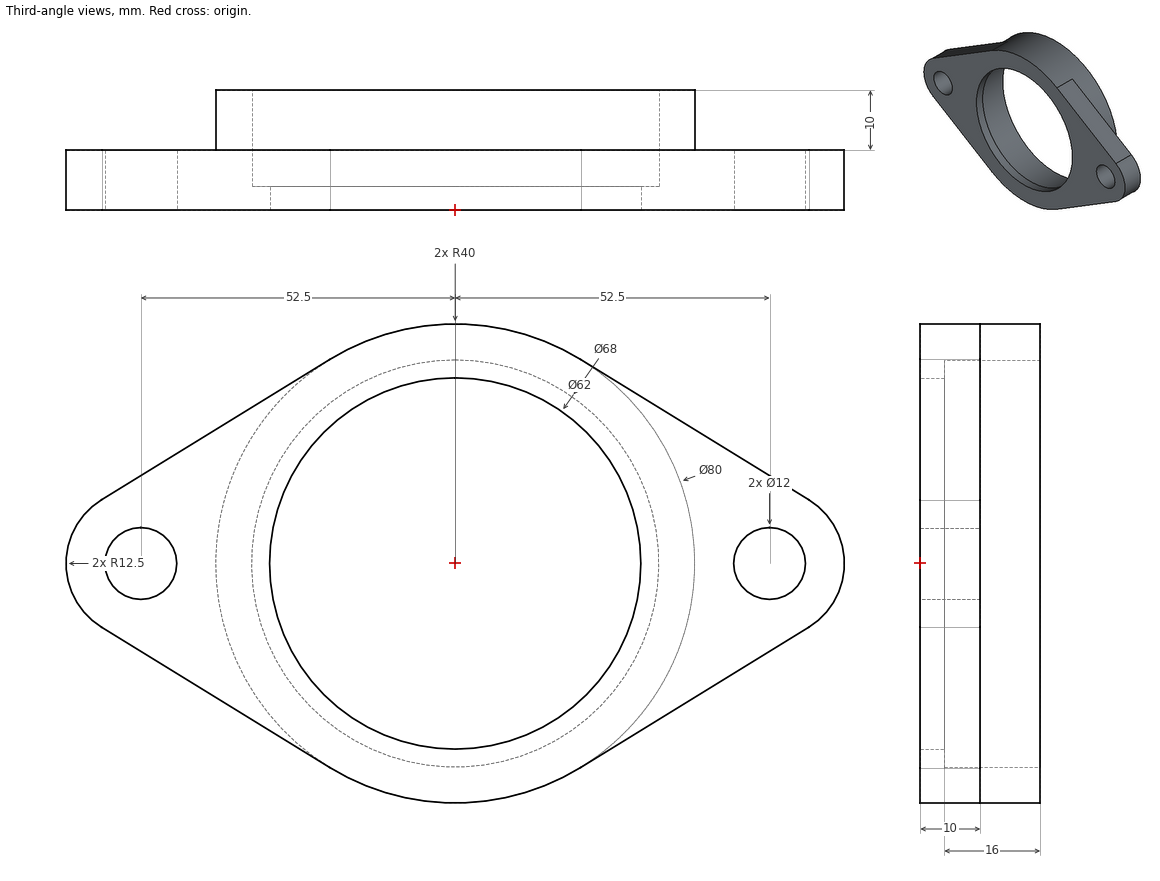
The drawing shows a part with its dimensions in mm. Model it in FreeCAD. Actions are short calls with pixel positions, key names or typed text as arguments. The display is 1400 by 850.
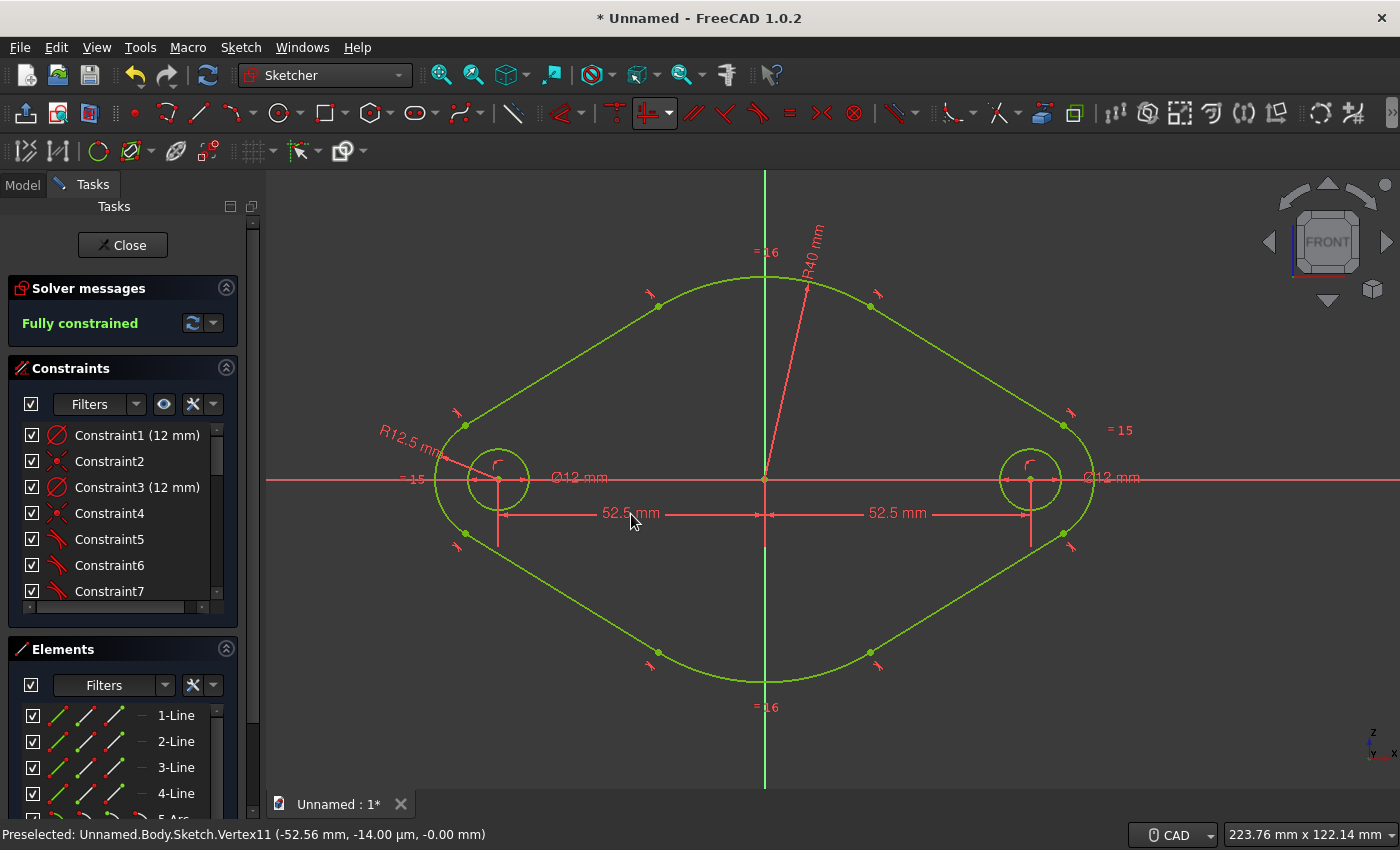
click(123, 245)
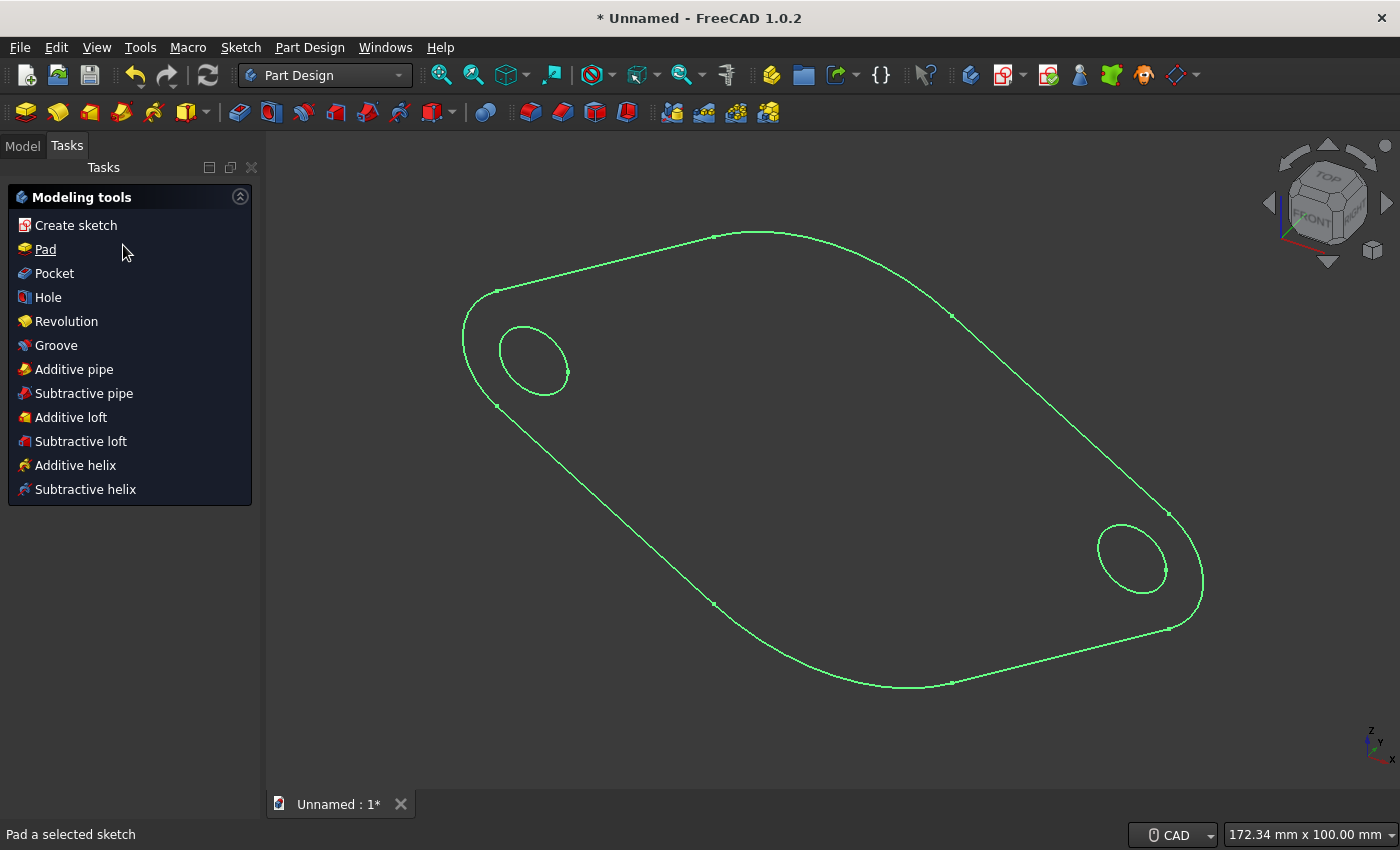
click(26, 112)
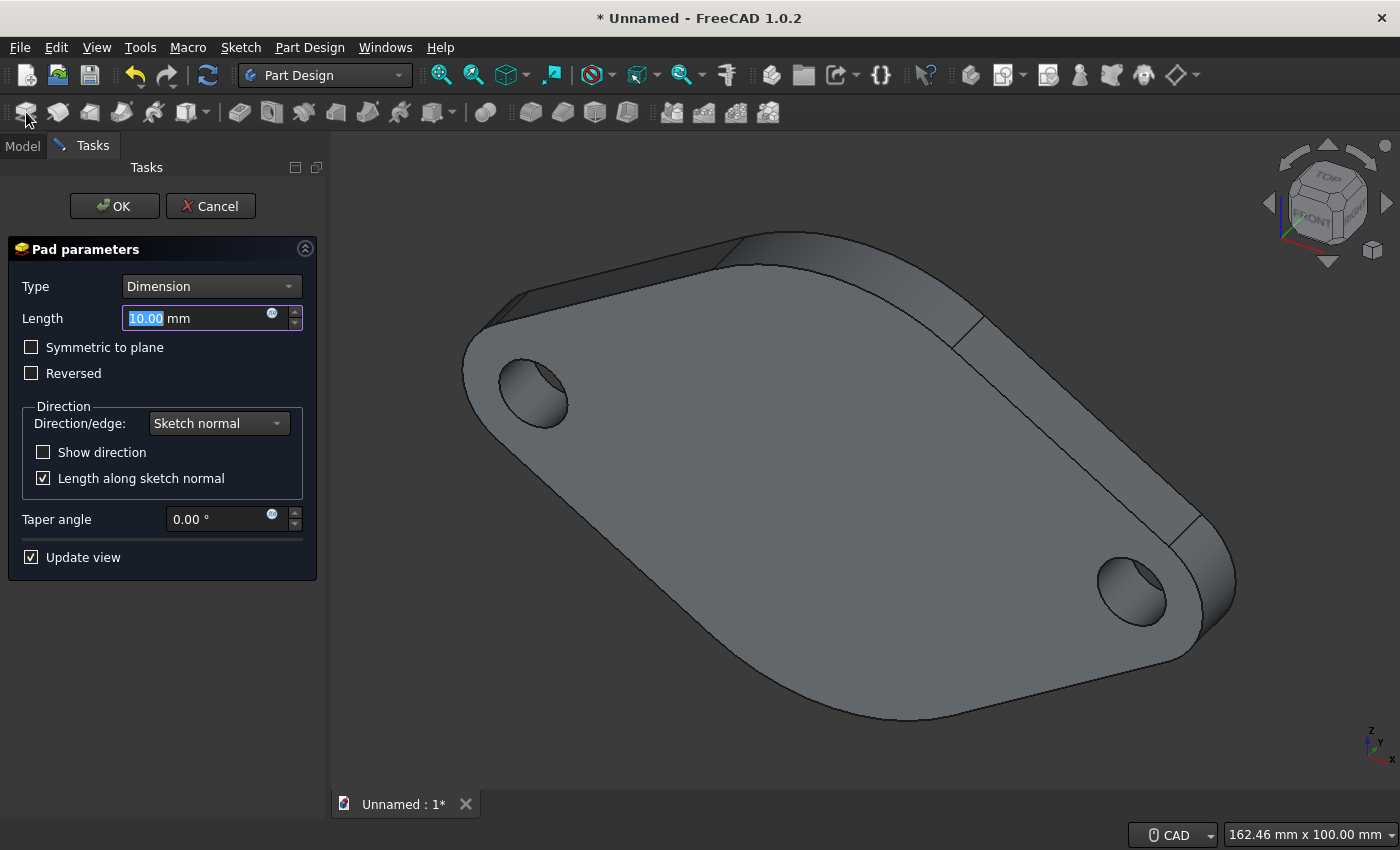
text(10)
key(Tab)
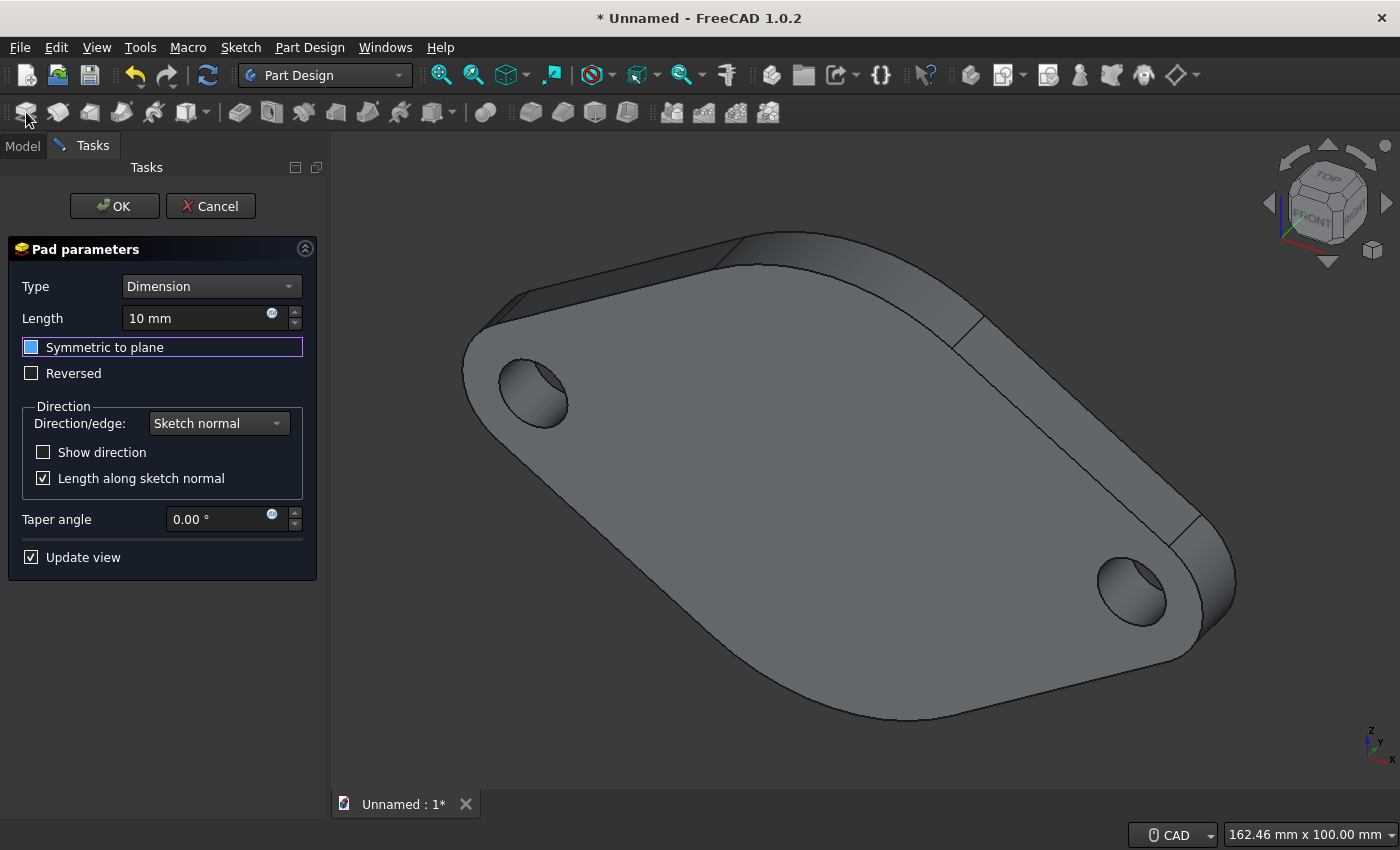
click(30, 373)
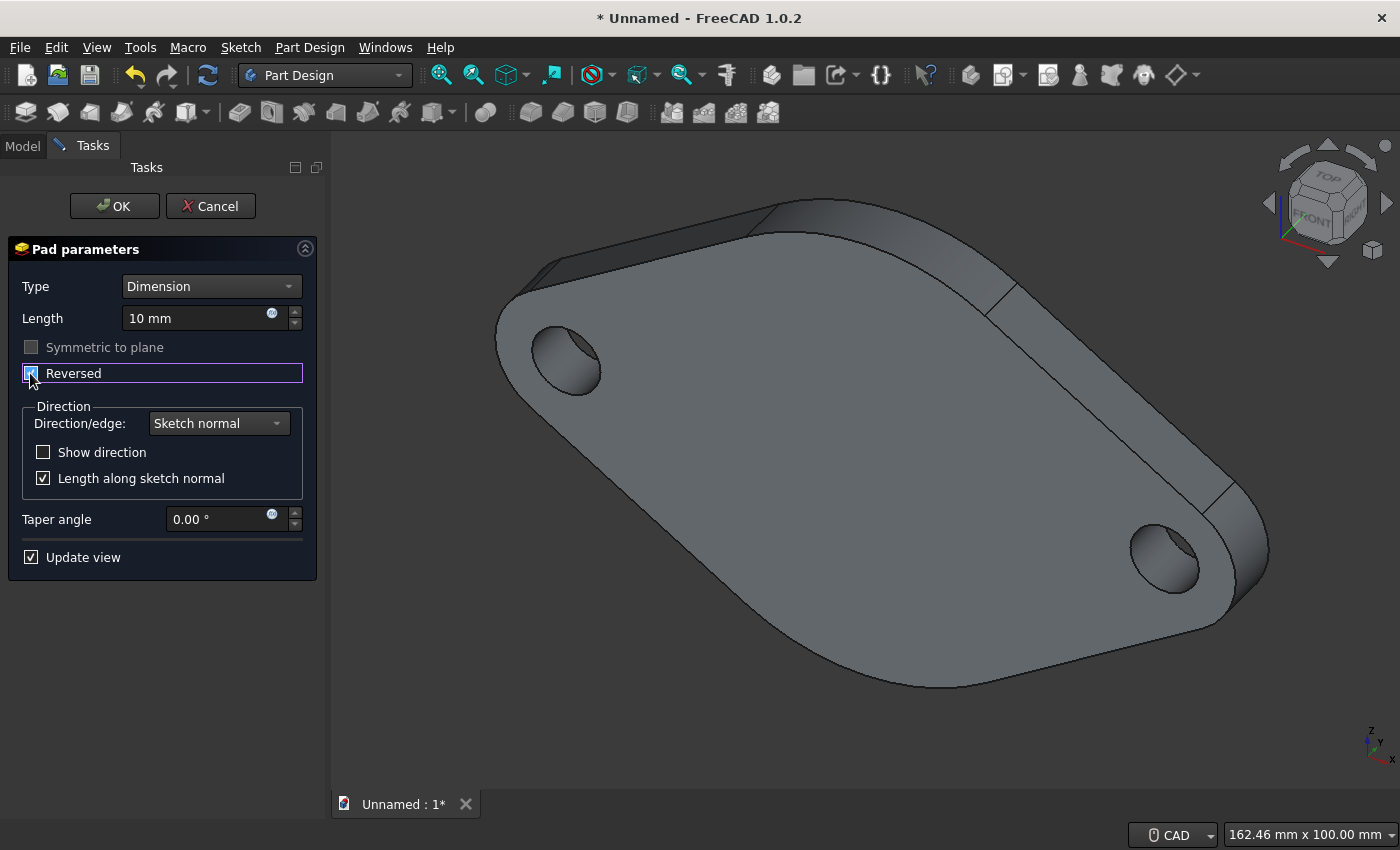
click(115, 206)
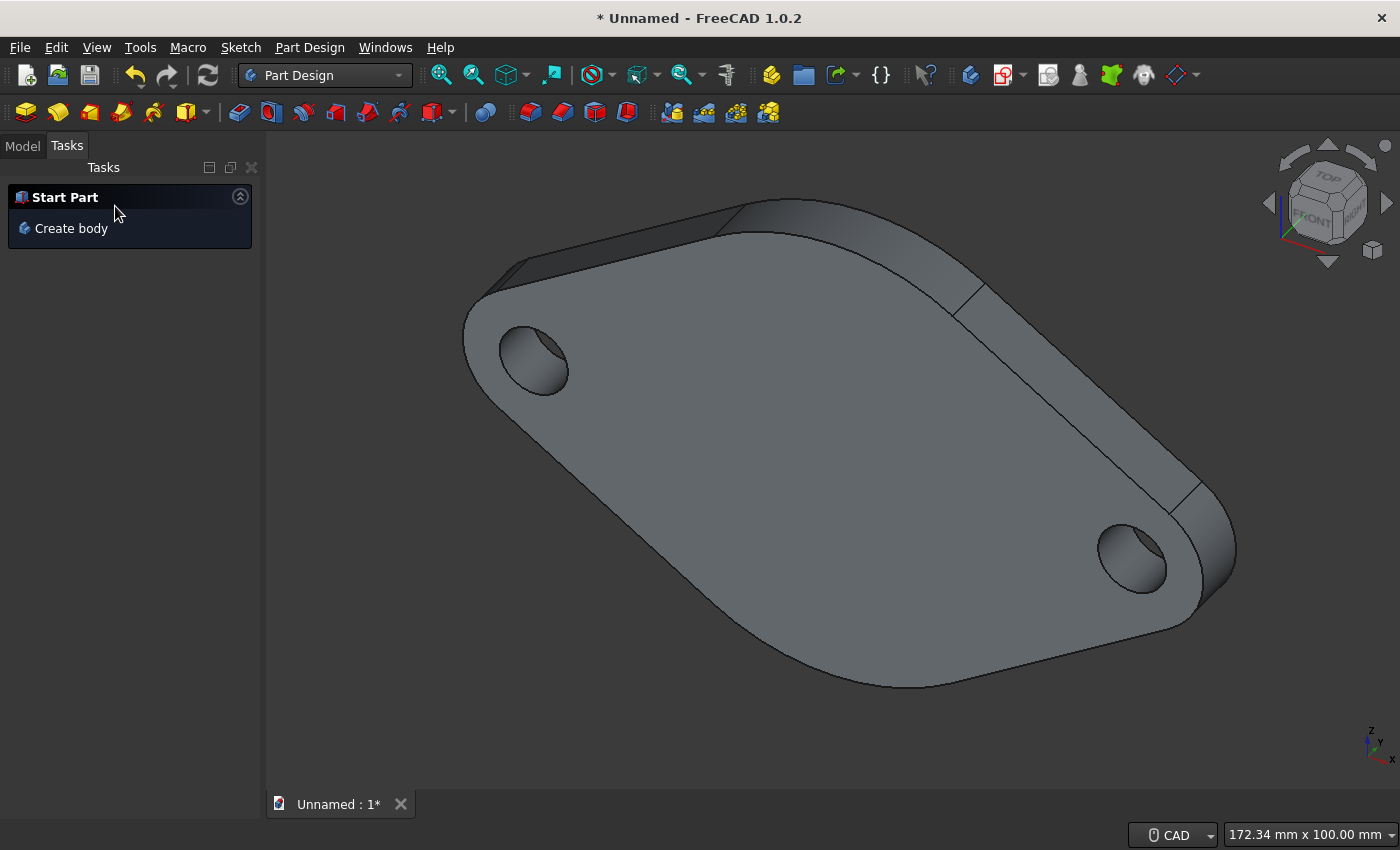
click(442, 76)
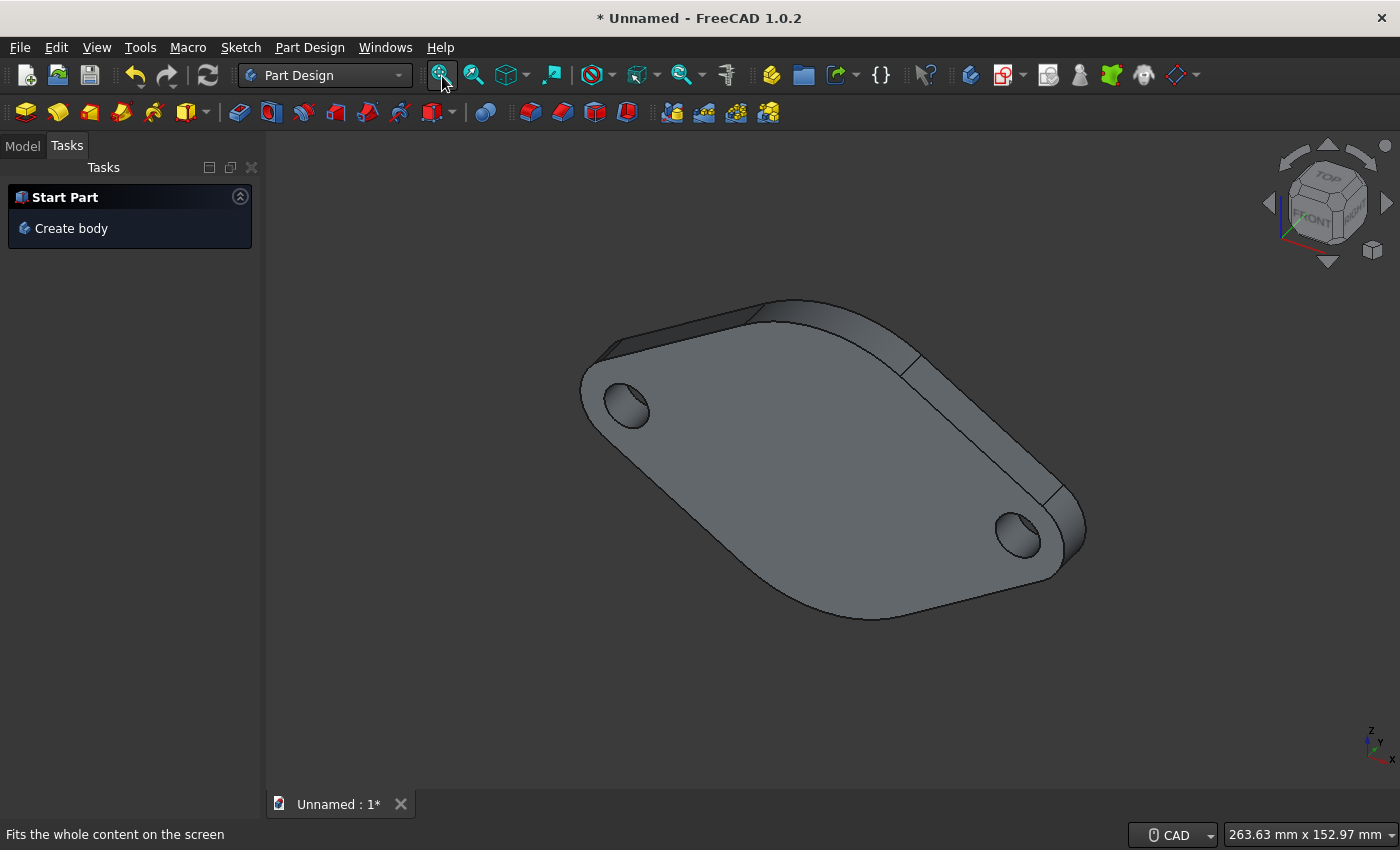
key(4)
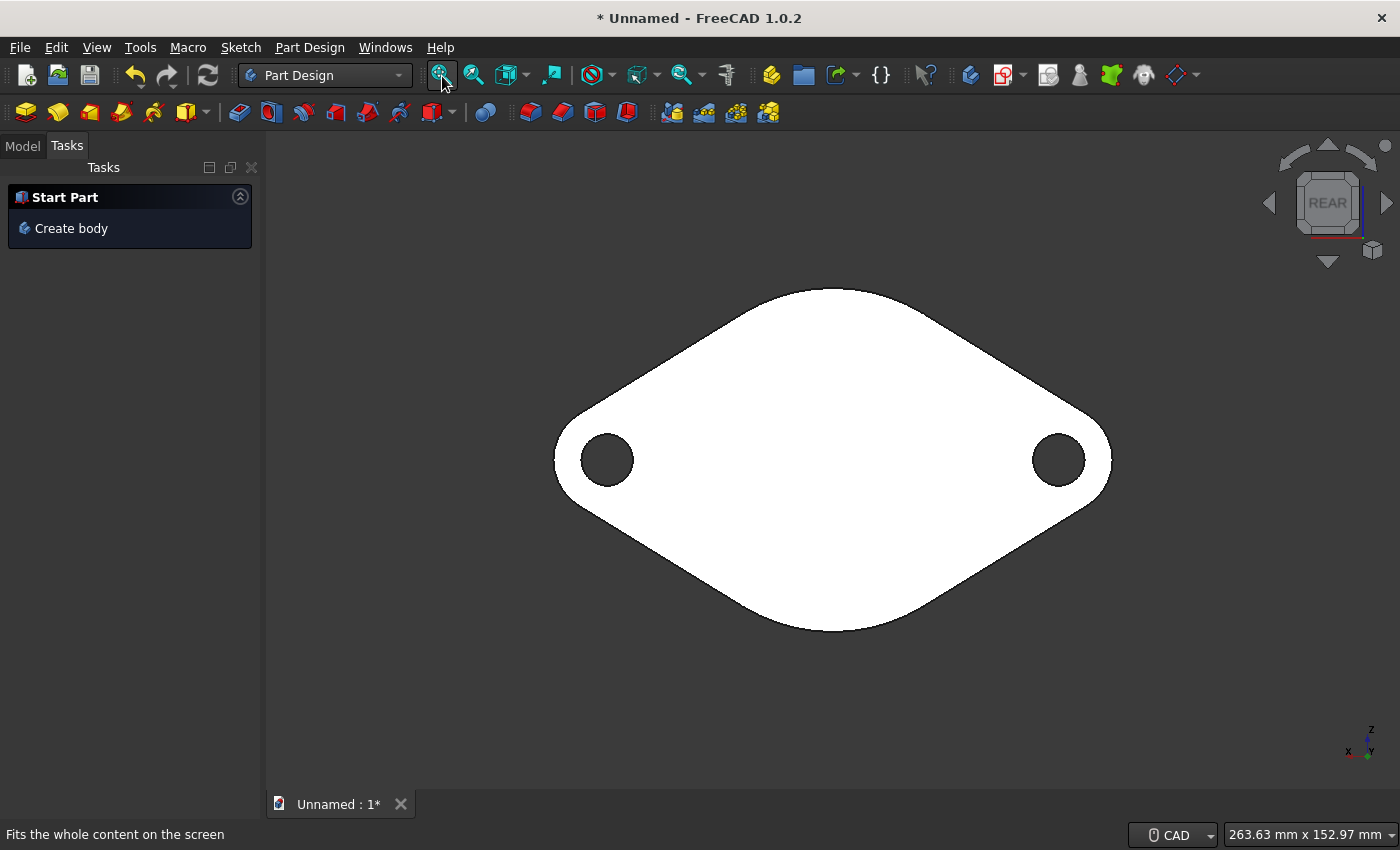
click(833, 459)